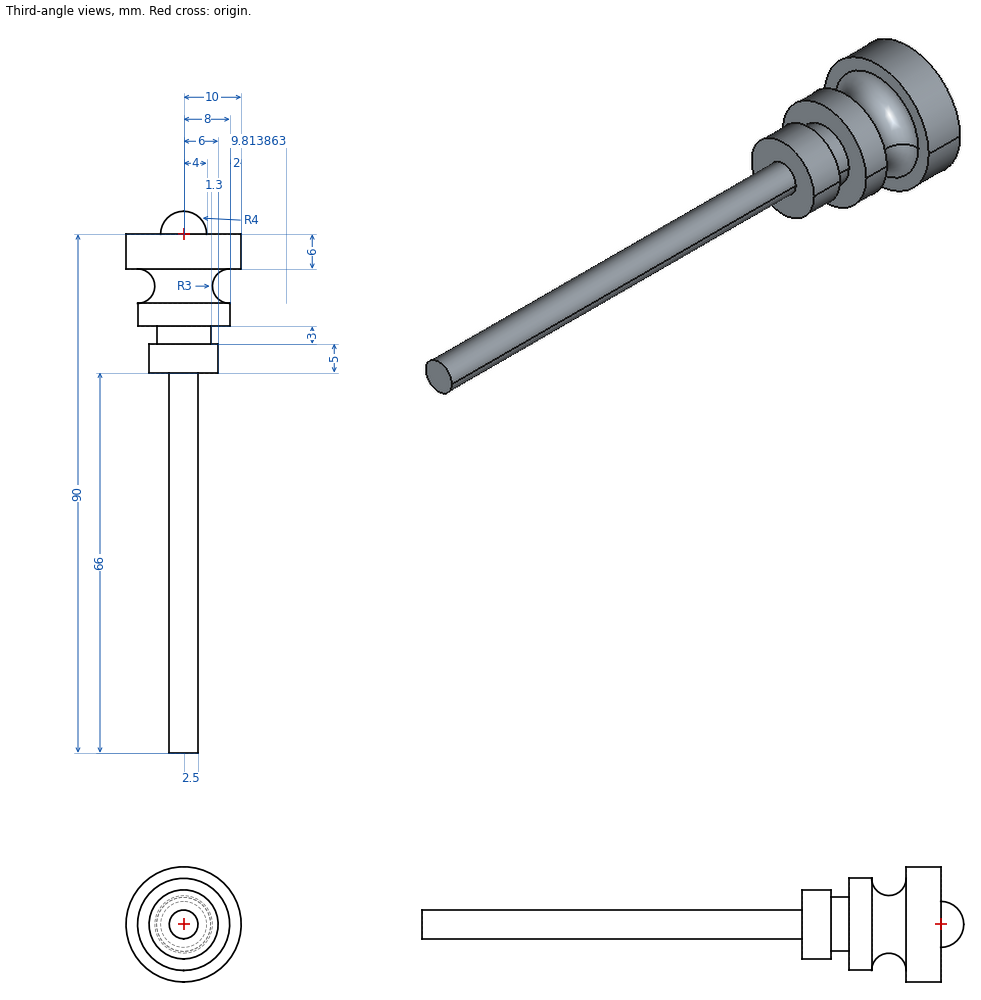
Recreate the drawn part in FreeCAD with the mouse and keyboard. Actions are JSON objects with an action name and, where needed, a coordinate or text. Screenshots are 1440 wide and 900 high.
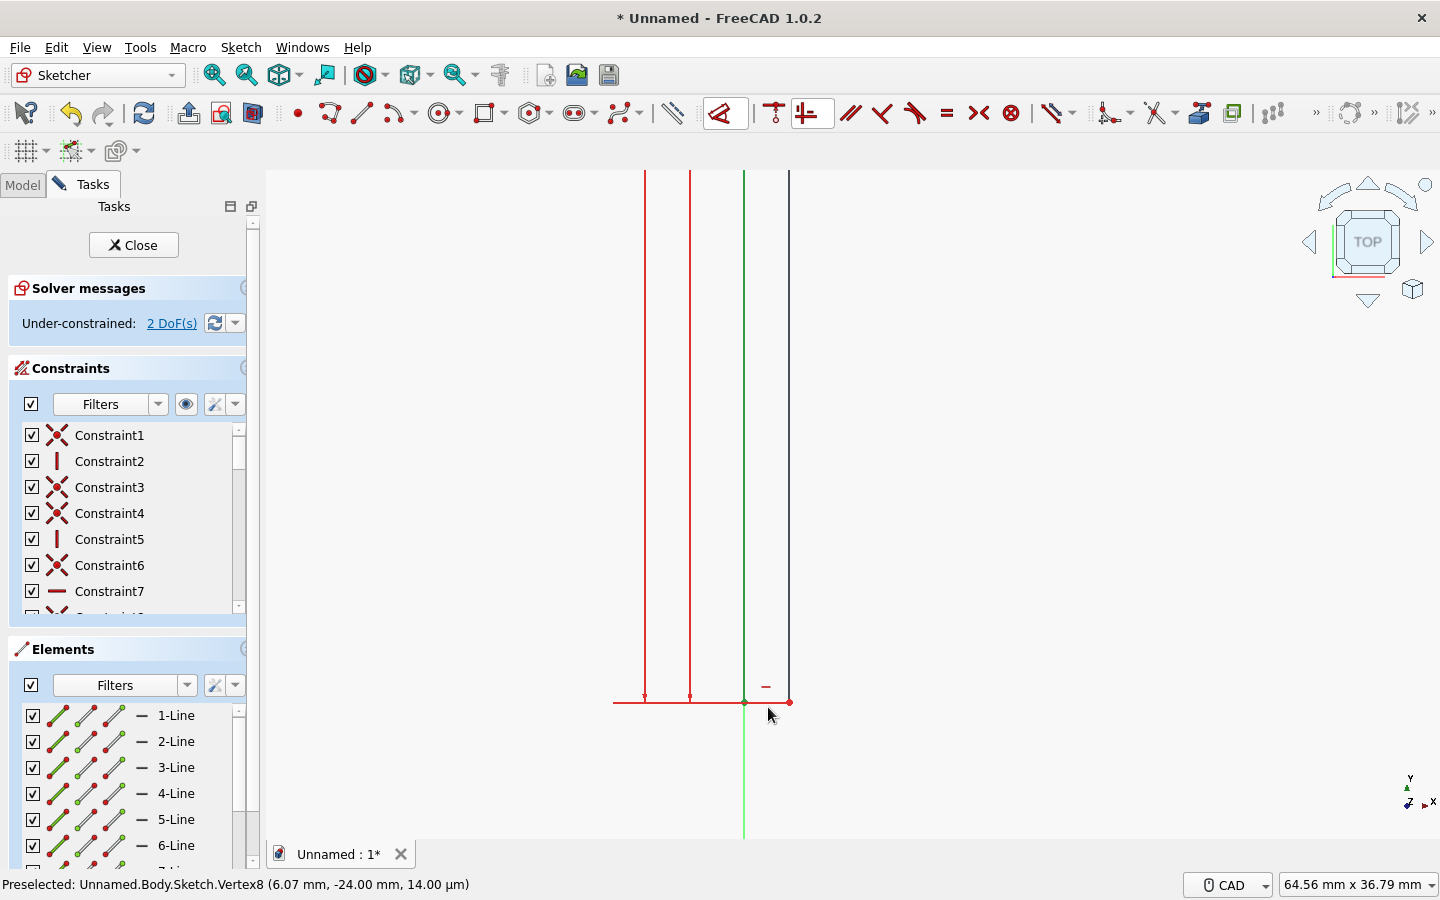
{"action": "left_click", "coordinate": [767, 703]}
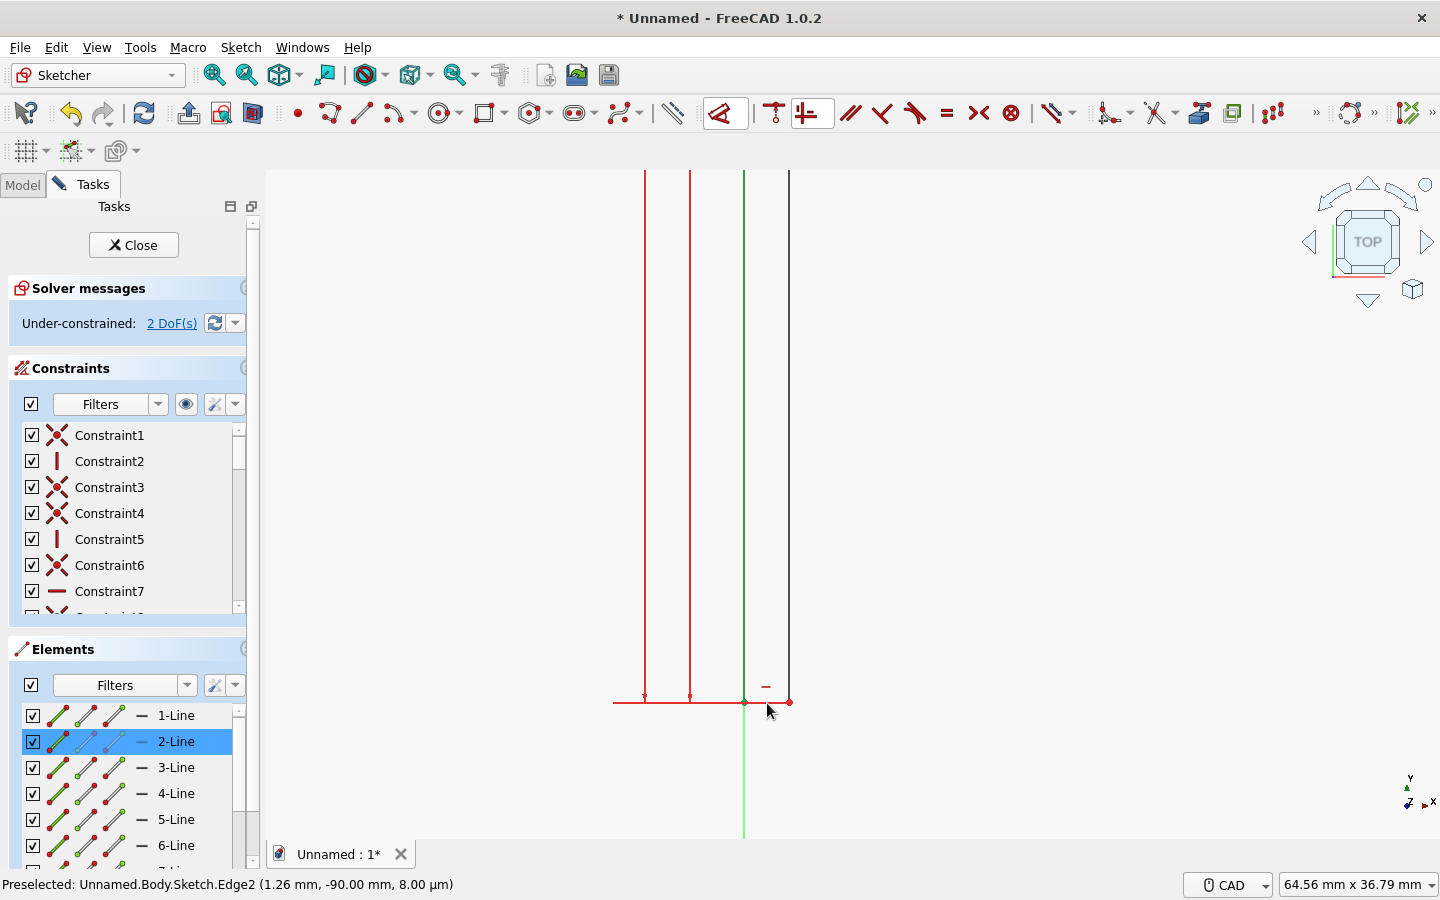
{"action": "key", "text": "l"}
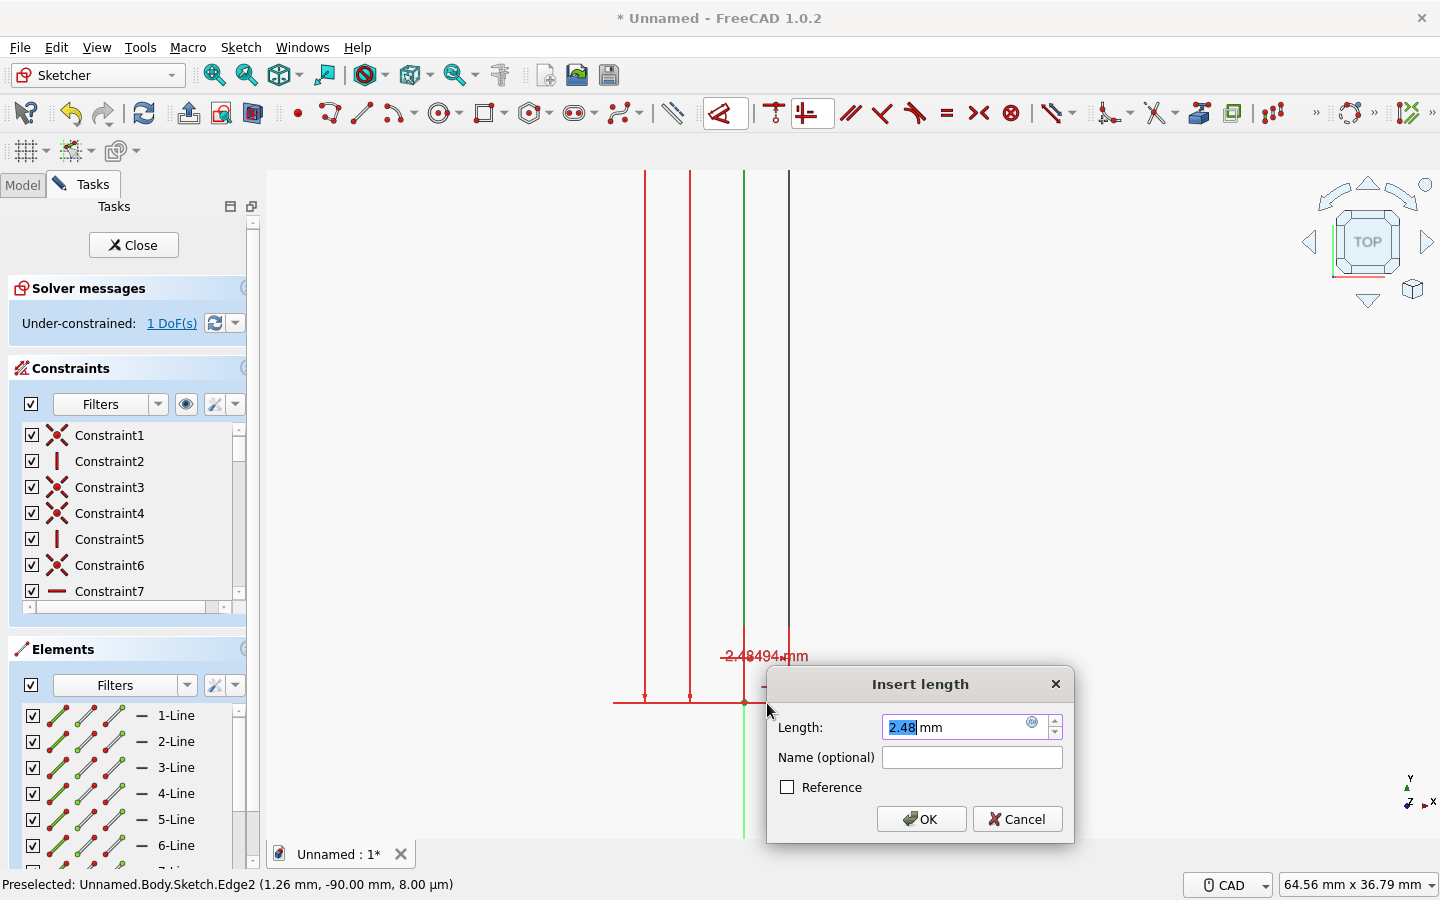
{"action": "type", "text": "2.5"}
{"action": "key", "text": "Return"}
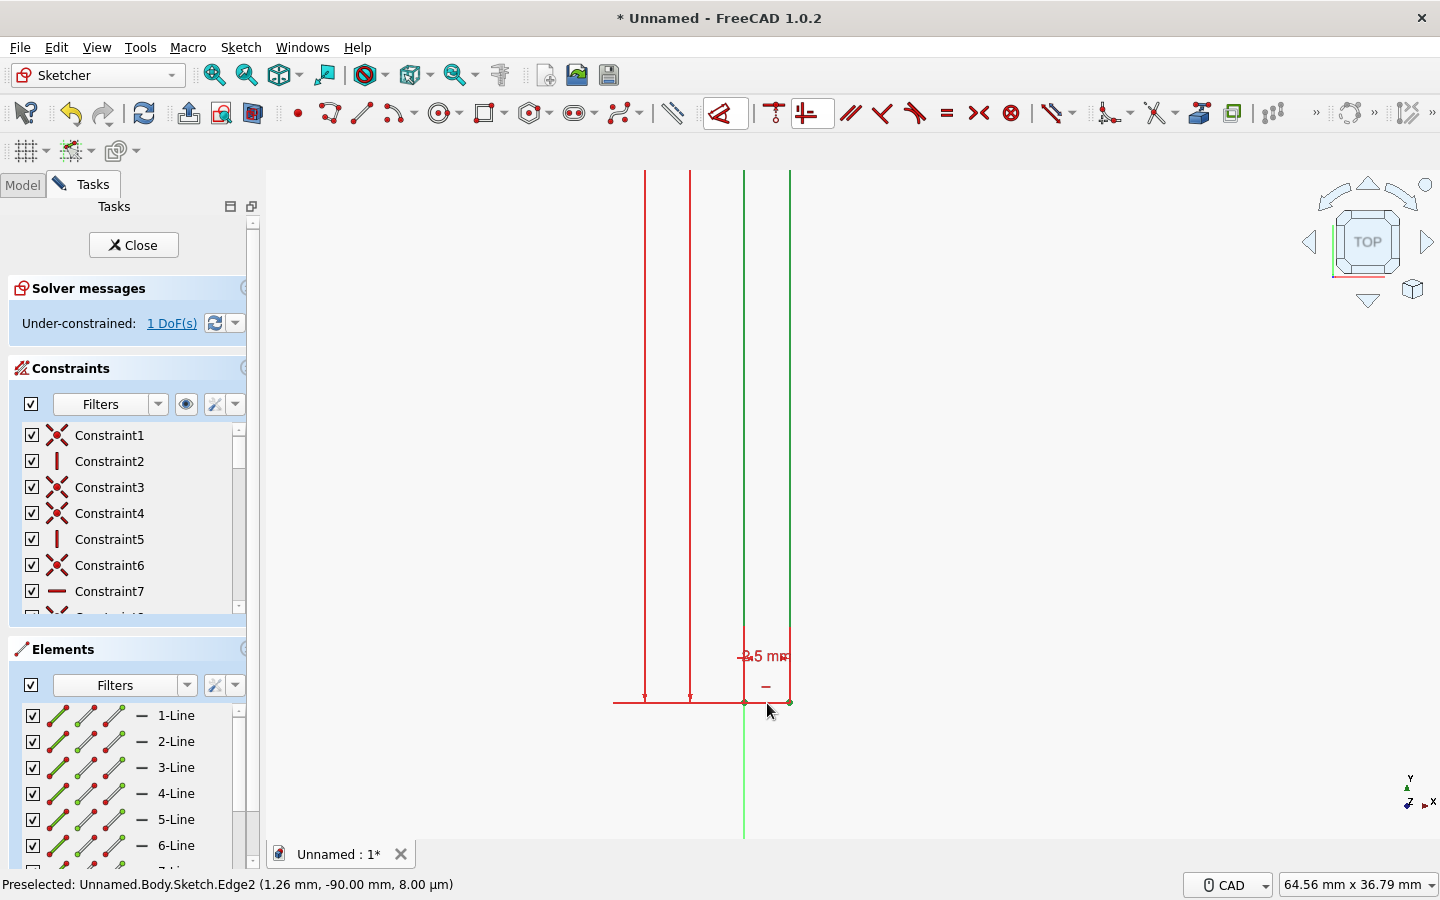
{"action": "scroll", "coordinate": [768, 707], "scroll_direction": "down", "scroll_amount": 7}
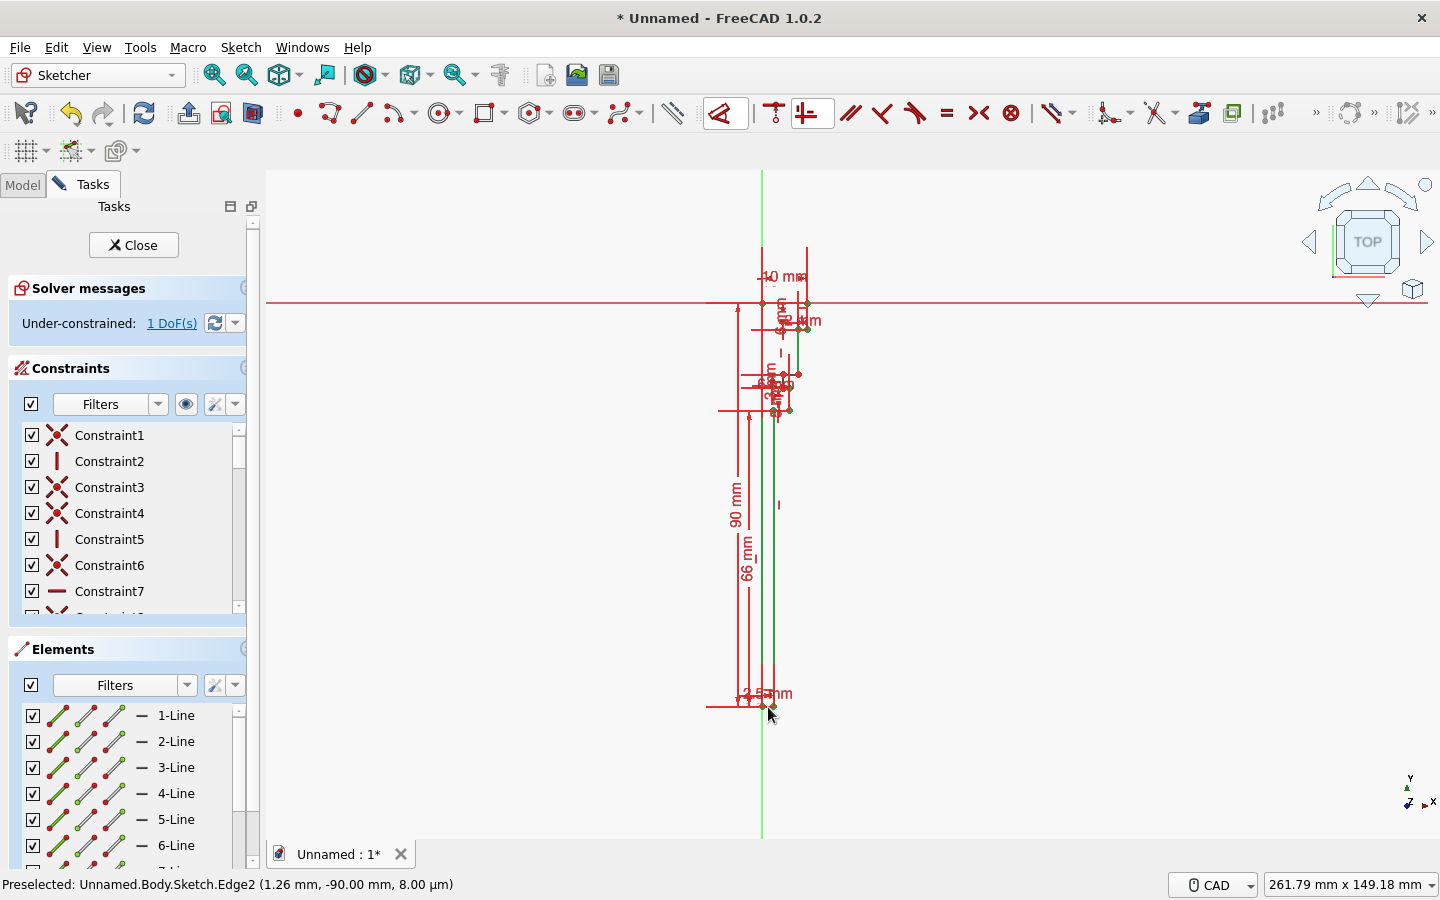
{"action": "scroll", "coordinate": [787, 388], "scroll_direction": "up", "scroll_amount": 10}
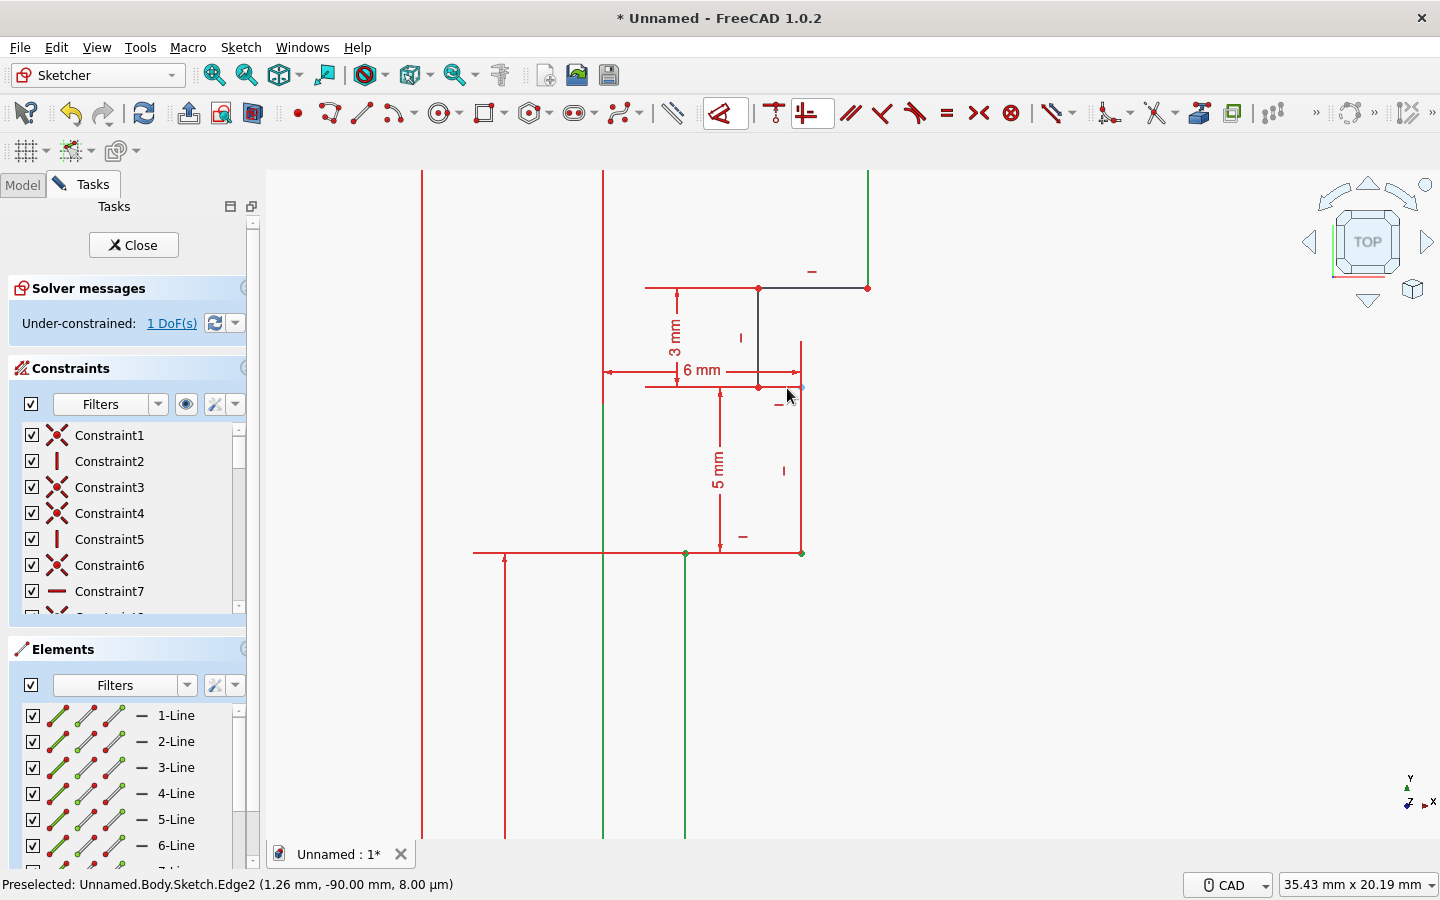
{"action": "left_click", "coordinate": [784, 387]}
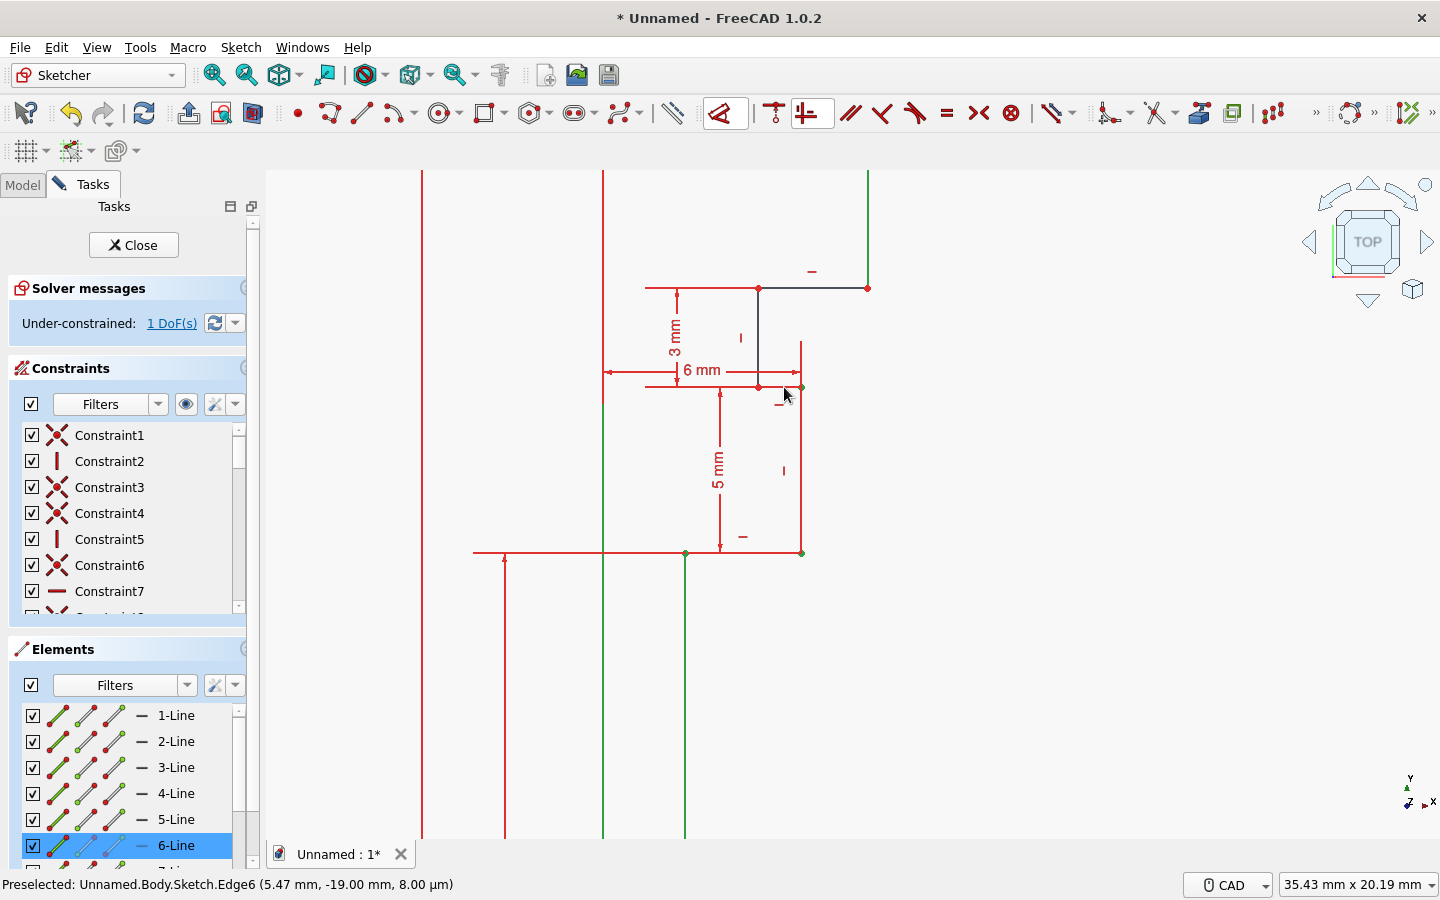
{"action": "key", "text": "l"}